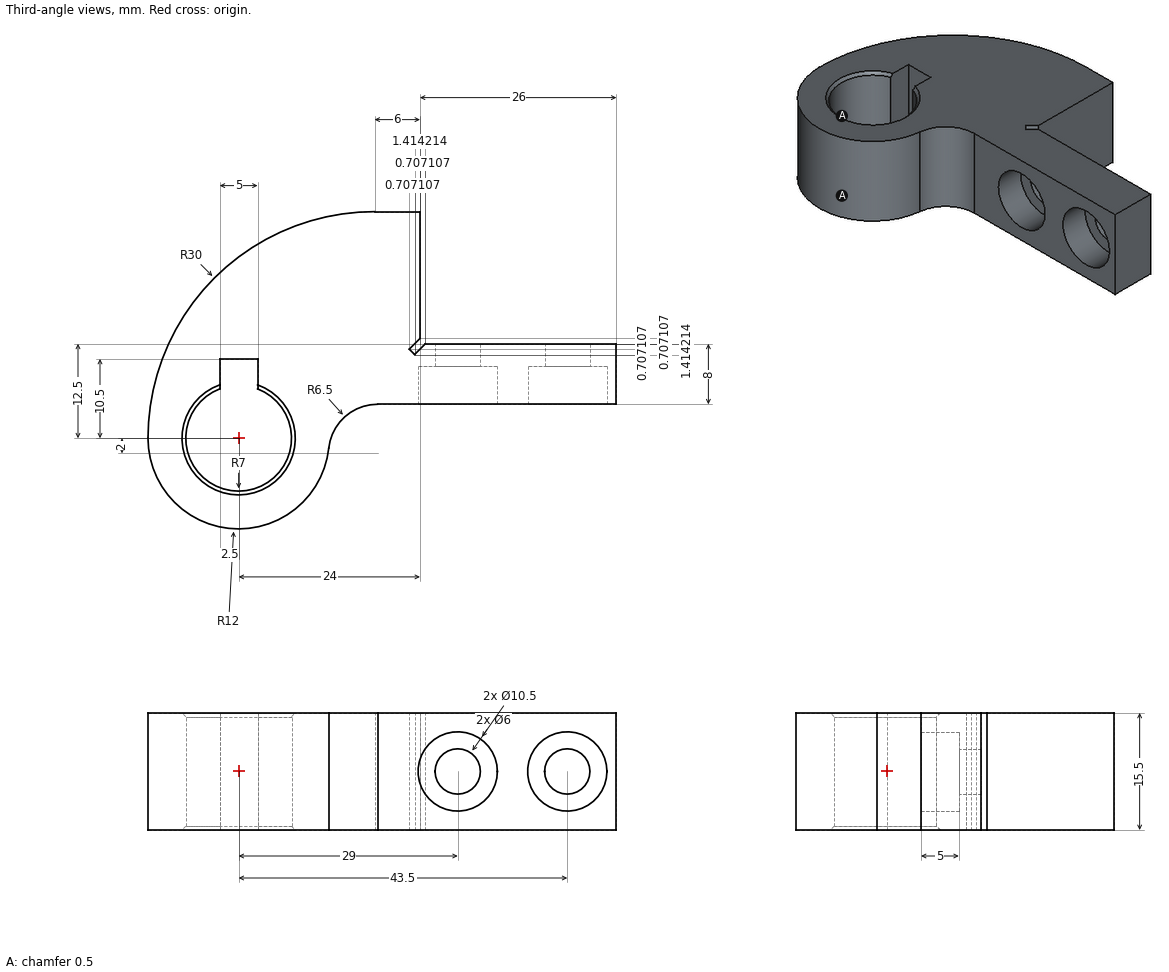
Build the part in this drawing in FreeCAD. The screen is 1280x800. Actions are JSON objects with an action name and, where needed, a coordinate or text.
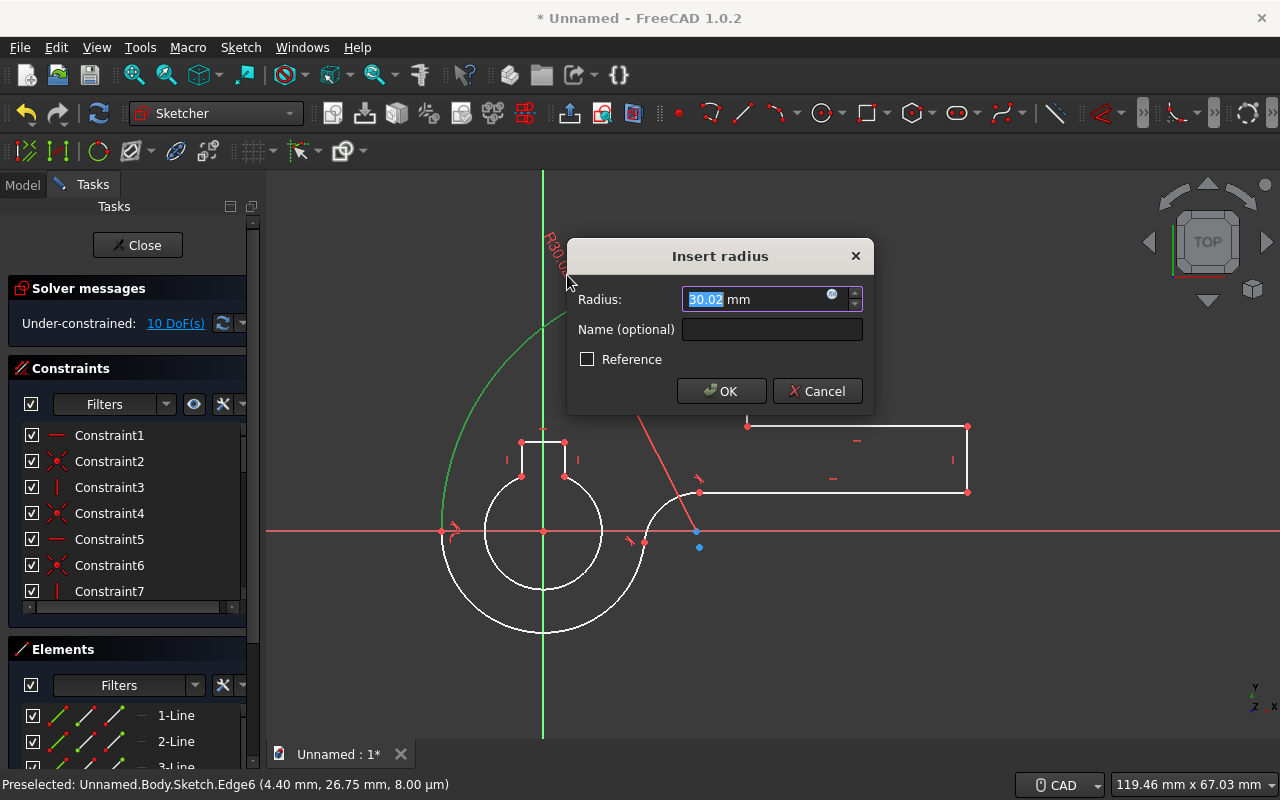
{"action": "type", "text": "30"}
{"action": "key", "text": "Return"}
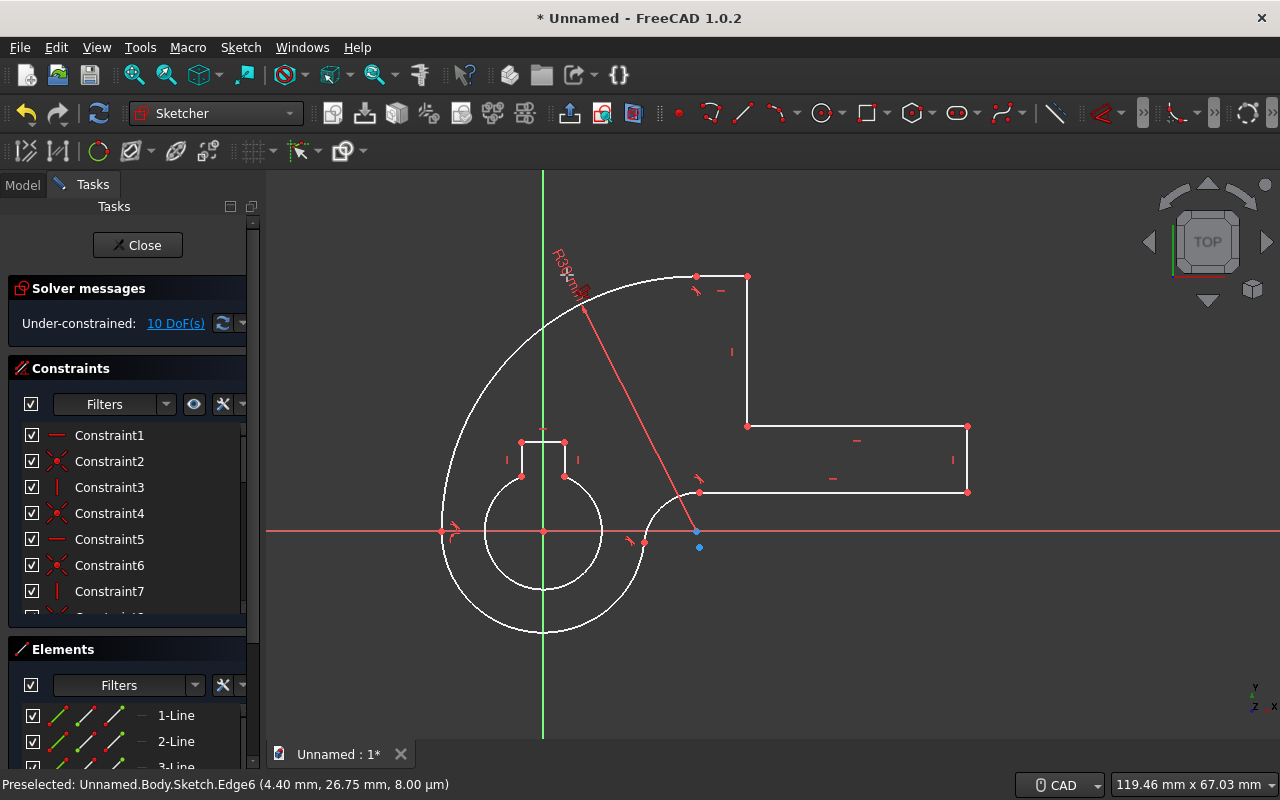
{"action": "left_click", "coordinate": [481, 611]}
{"action": "left_click", "coordinate": [461, 636]}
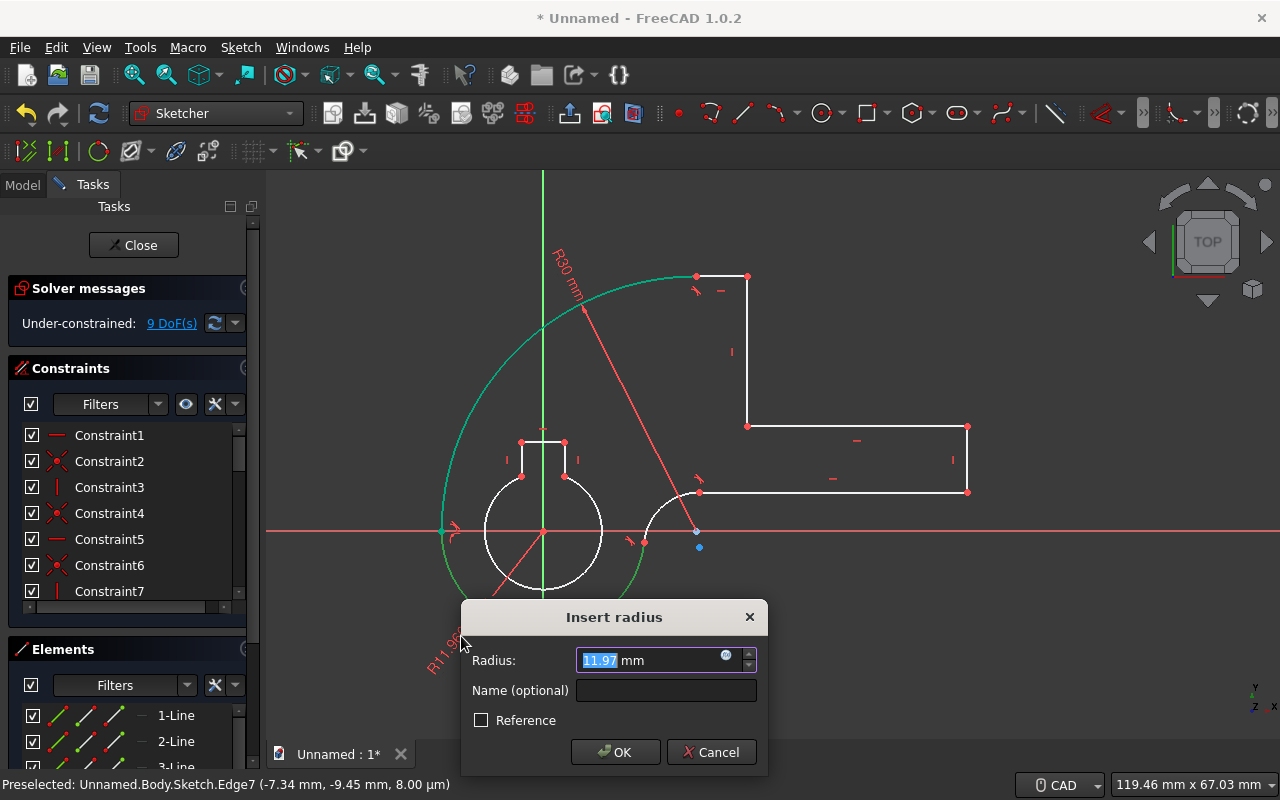
{"action": "type", "text": "12"}
{"action": "key", "text": "Return"}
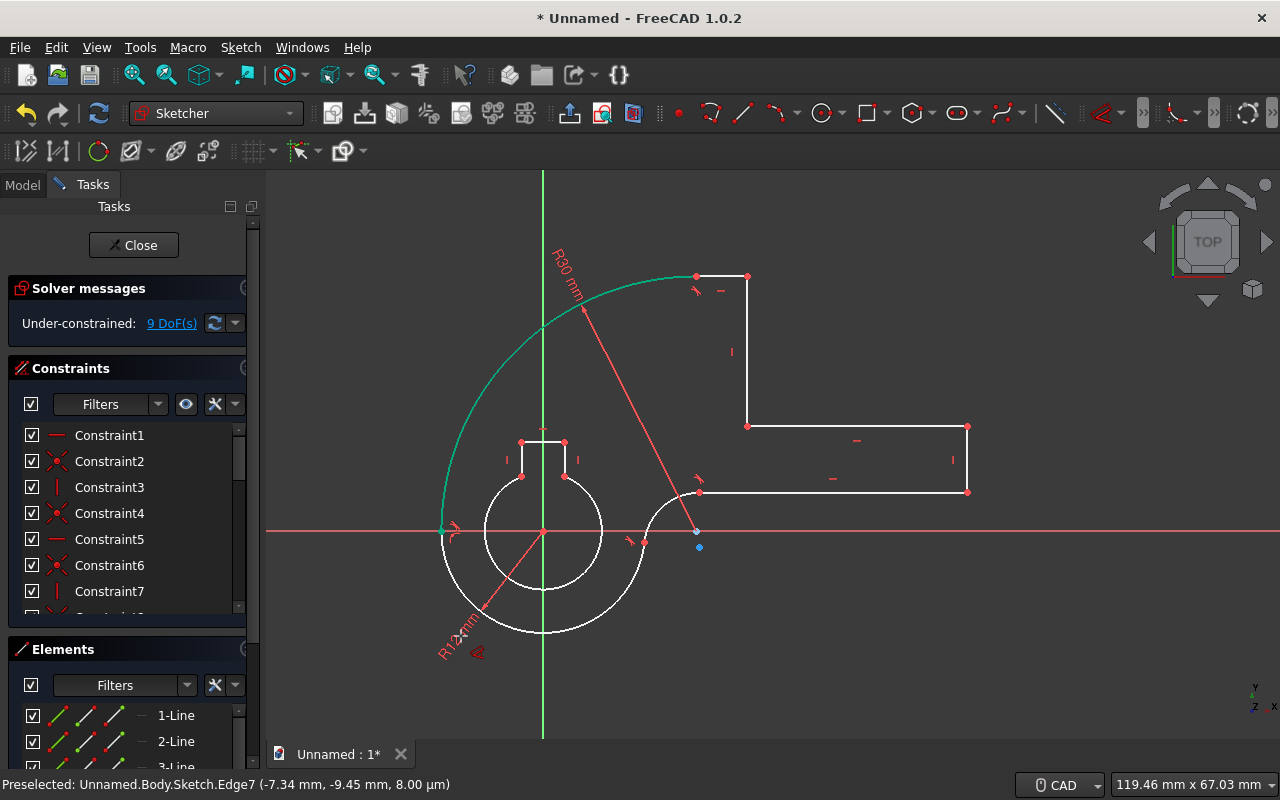
{"action": "left_click", "coordinate": [676, 498]}
{"action": "left_click", "coordinate": [662, 469]}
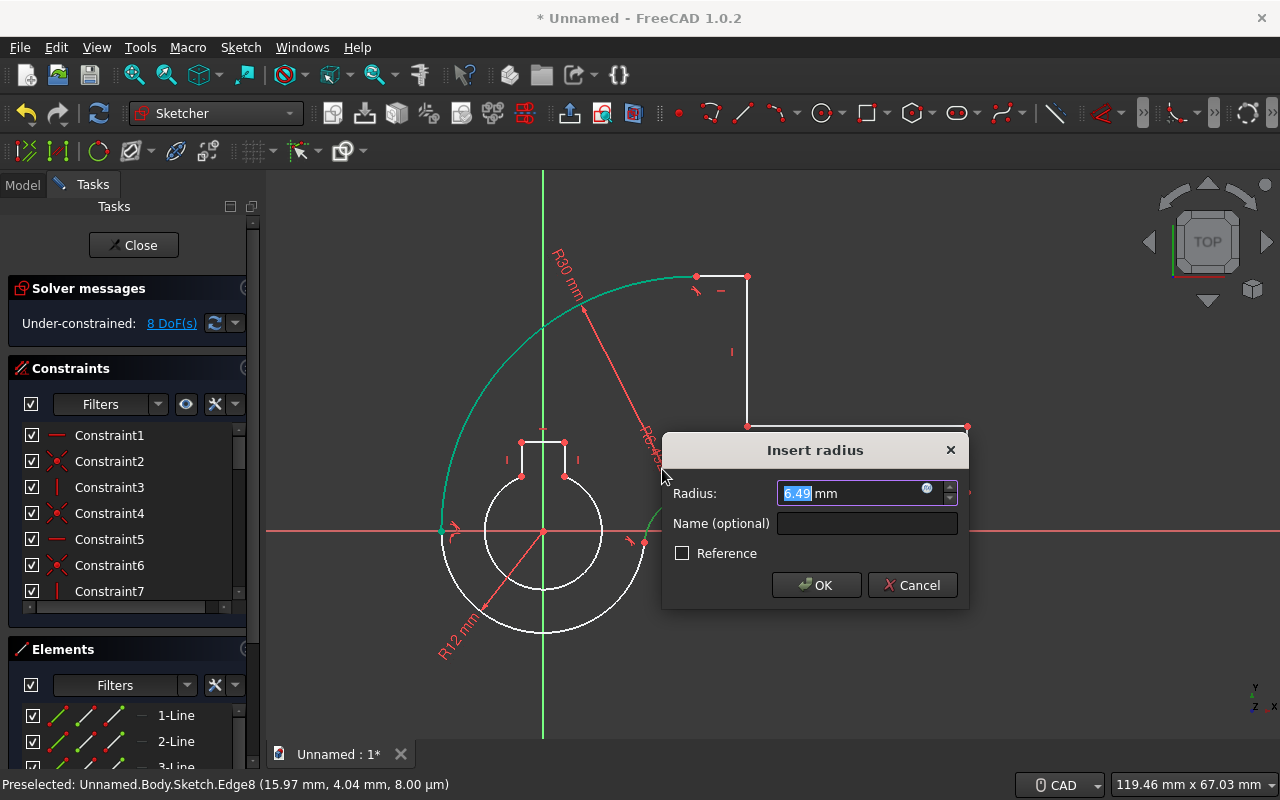
{"action": "type", "text": "6.5"}
{"action": "key", "text": "Return"}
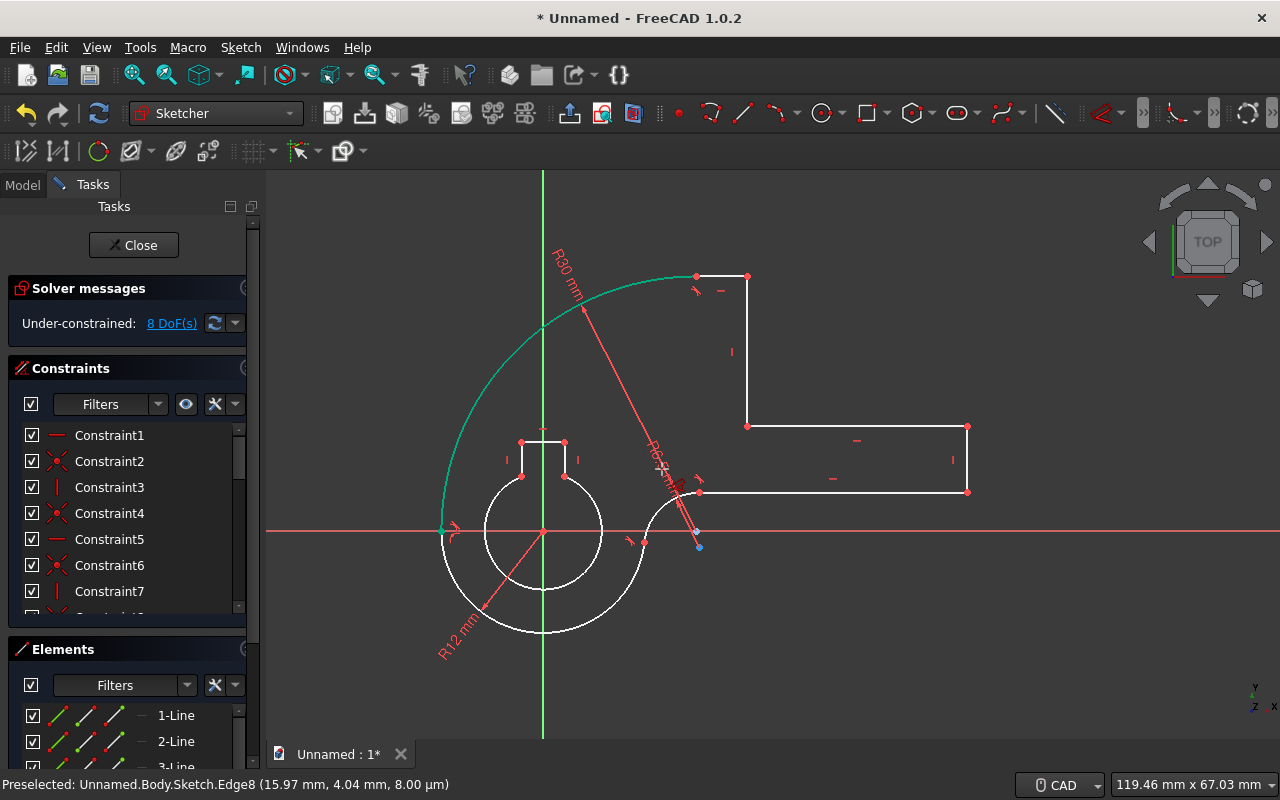
{"action": "left_click", "coordinate": [491, 557]}
{"action": "left_click", "coordinate": [466, 485]}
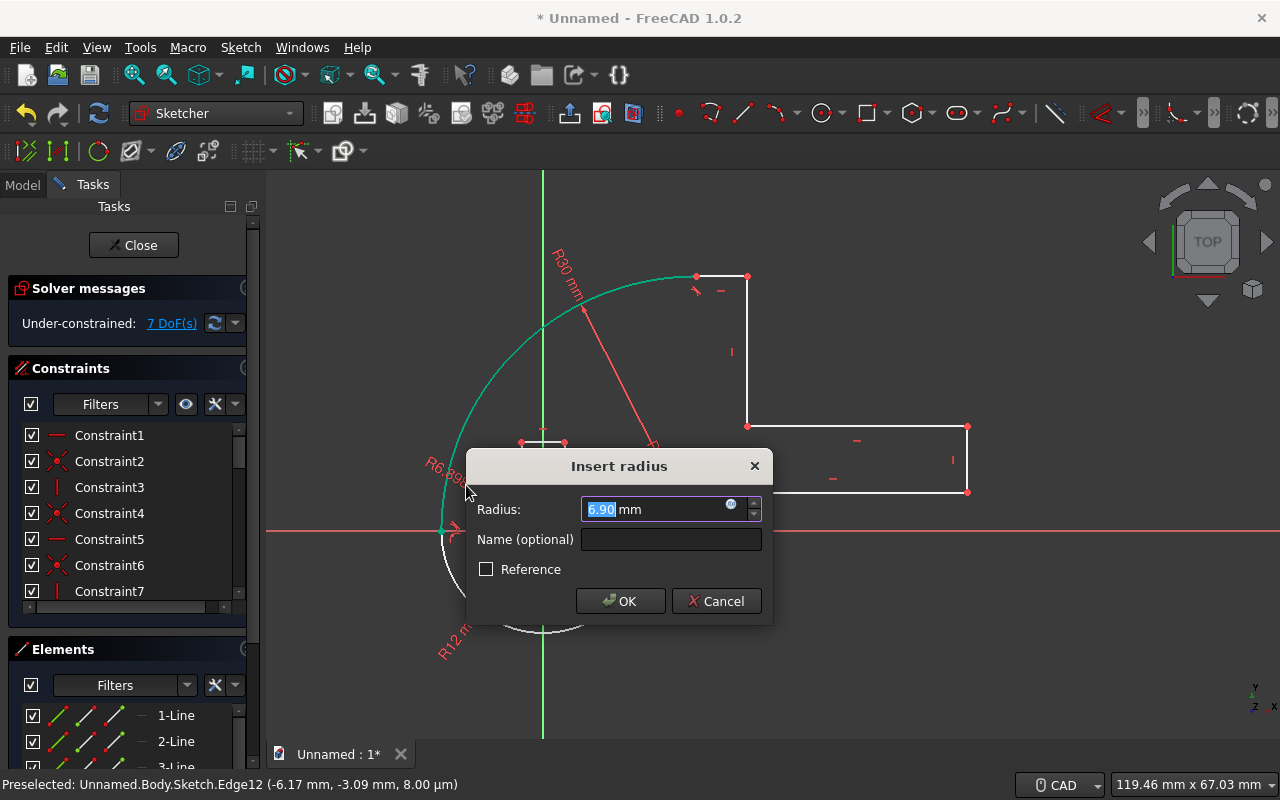
{"action": "type", "text": "7"}
{"action": "key", "text": "Return"}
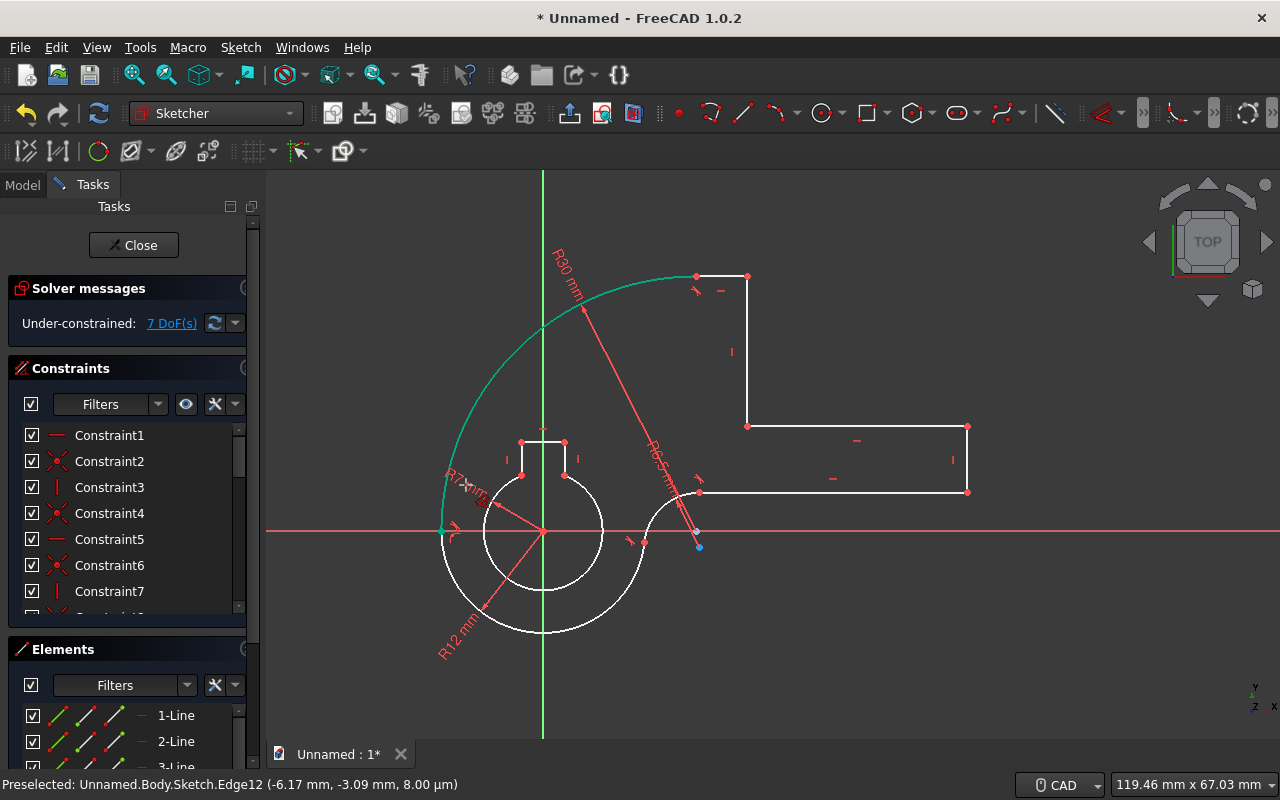
{"action": "left_click", "coordinate": [967, 473]}
{"action": "left_click", "coordinate": [1001, 459]}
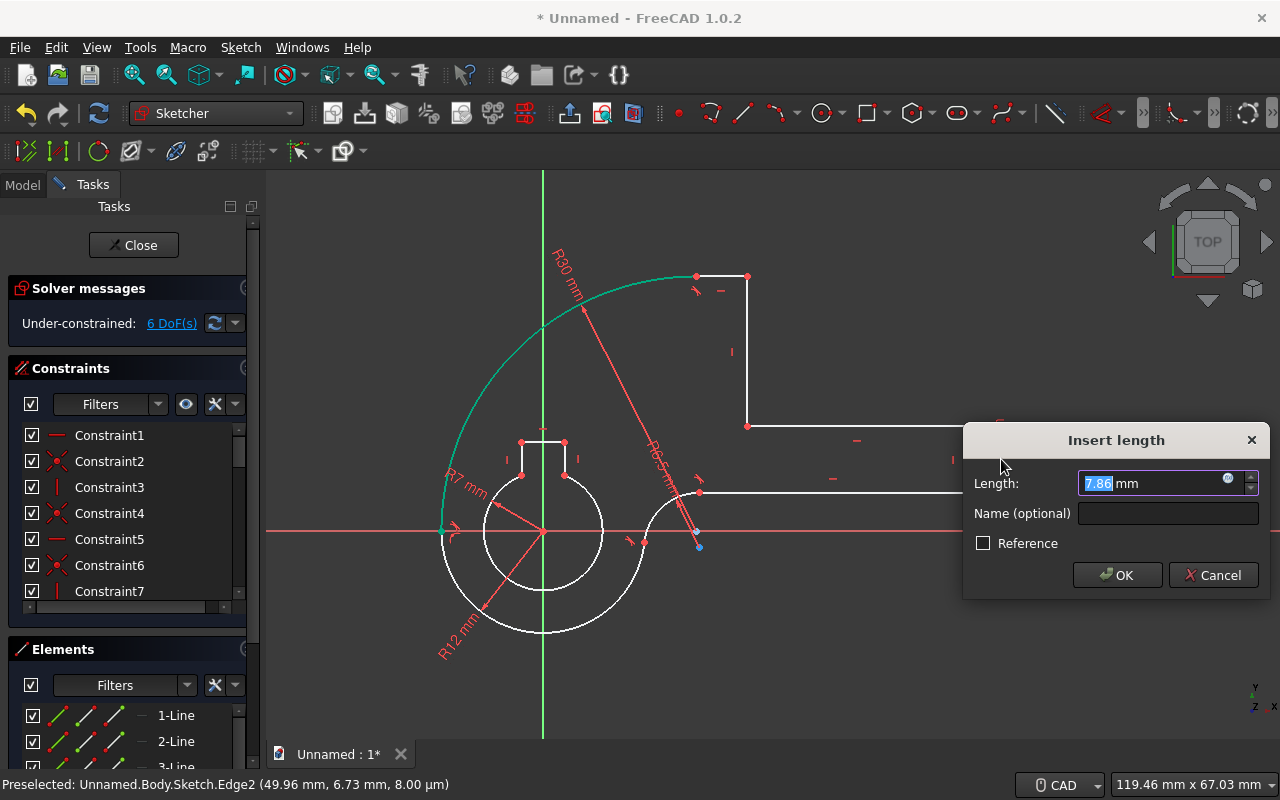
{"action": "type", "text": "8"}
{"action": "key", "text": "Return"}